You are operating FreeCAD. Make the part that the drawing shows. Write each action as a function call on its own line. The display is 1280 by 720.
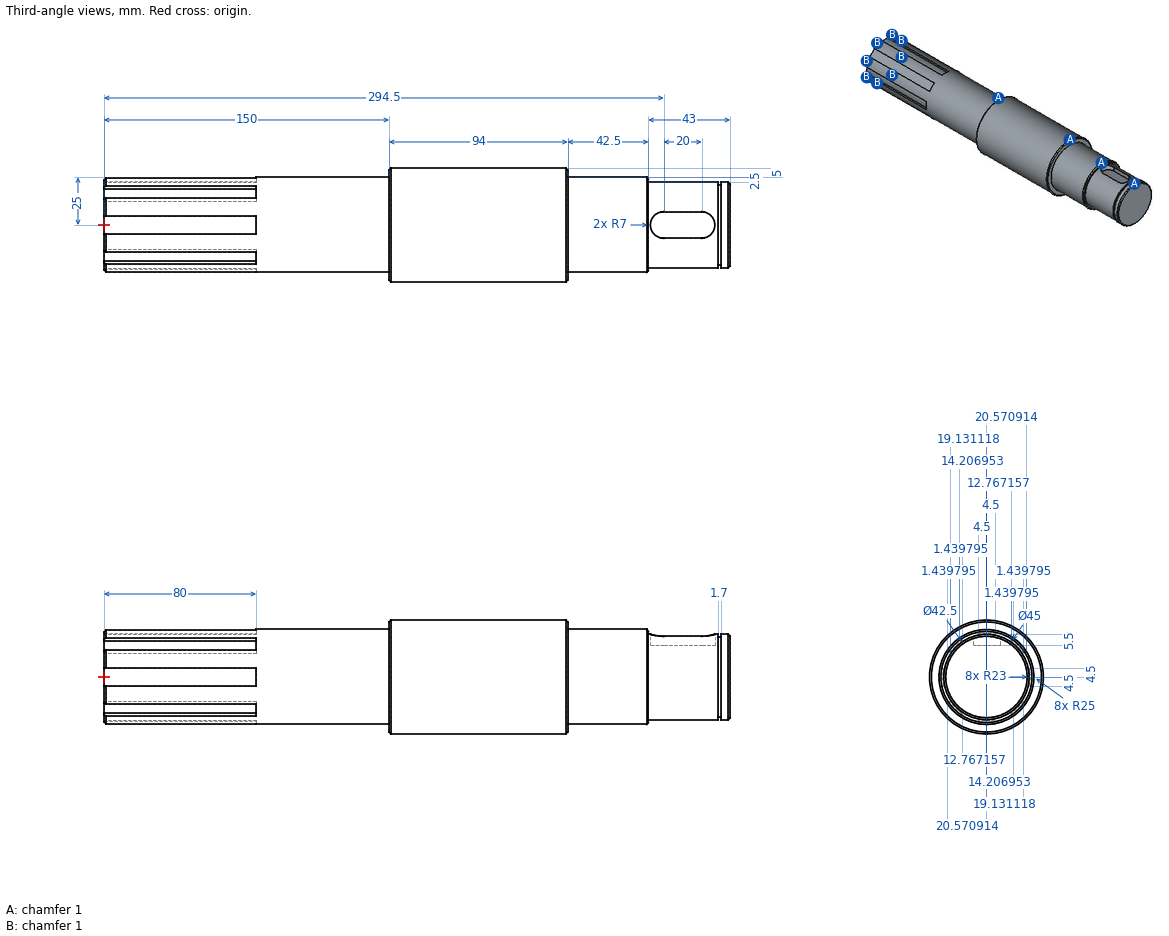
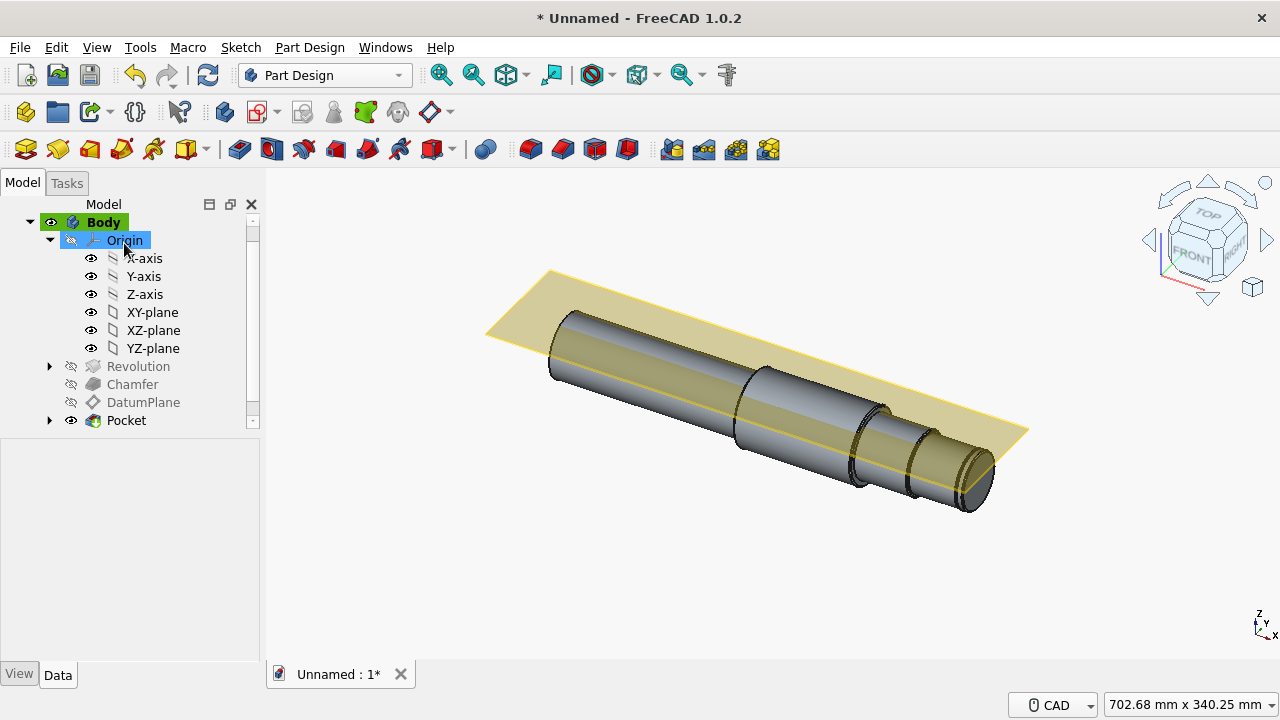
scroll(120, 326, down, 3)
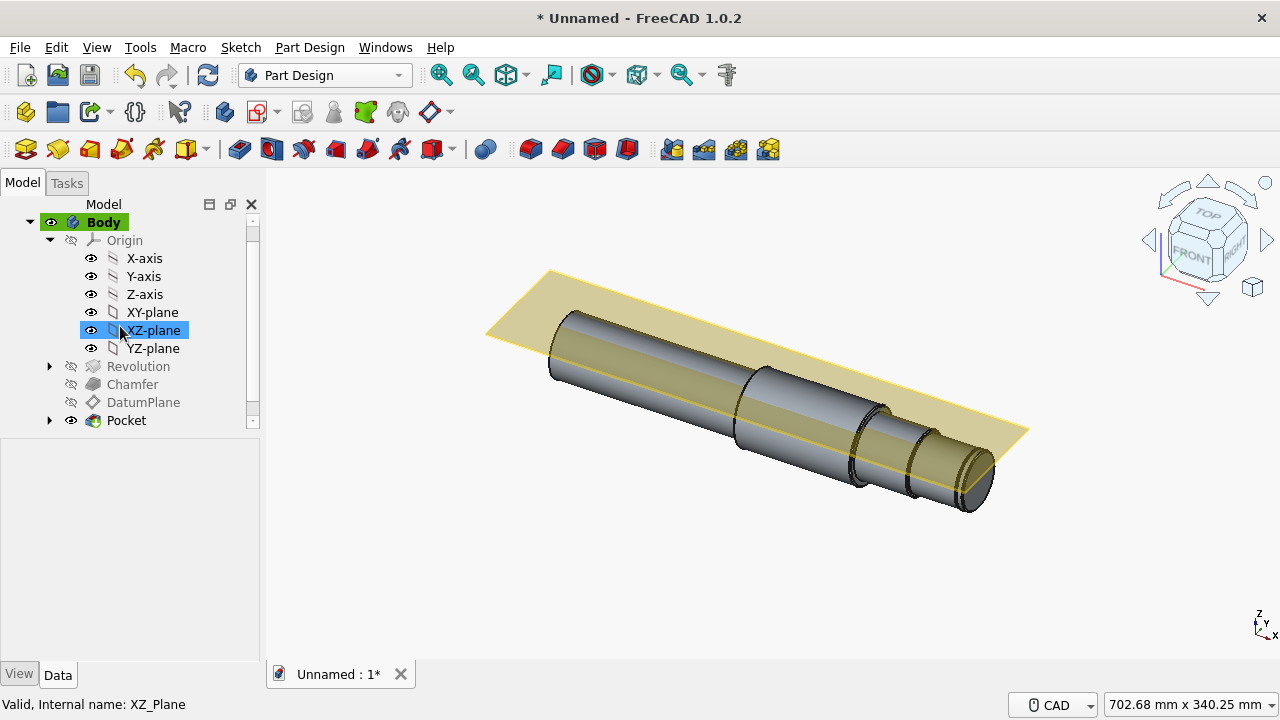
click(116, 420)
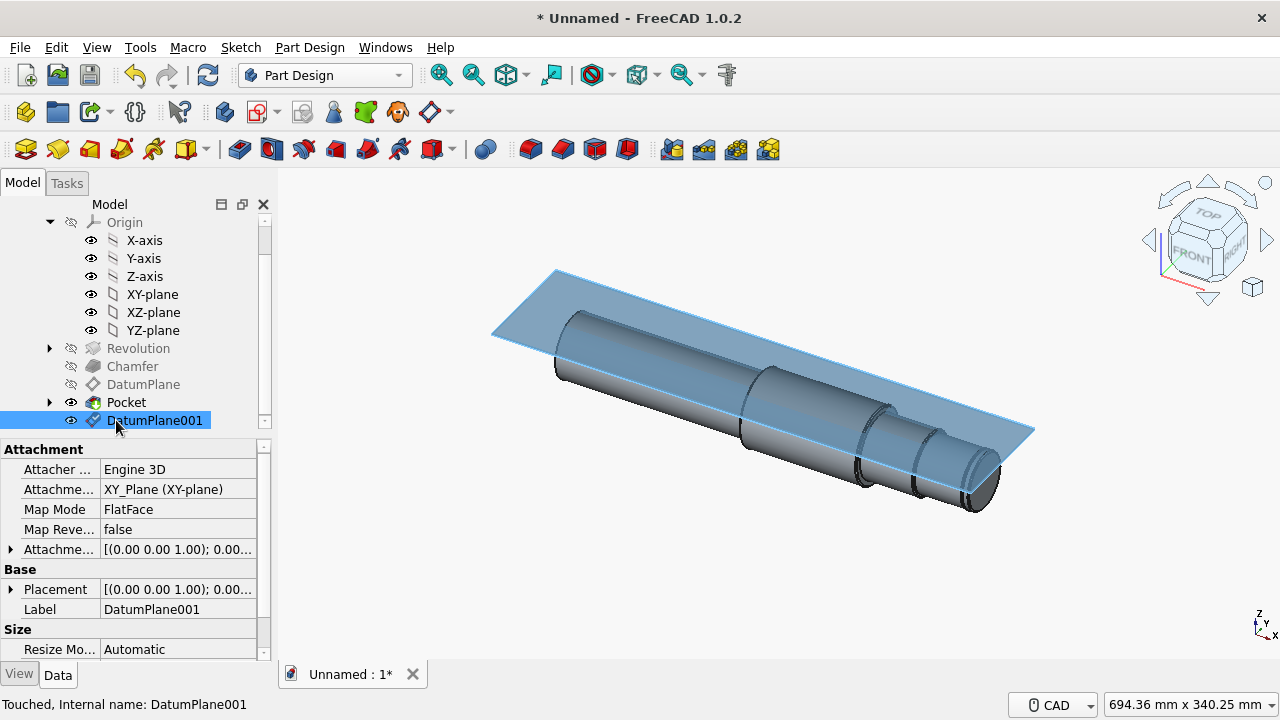
click(258, 112)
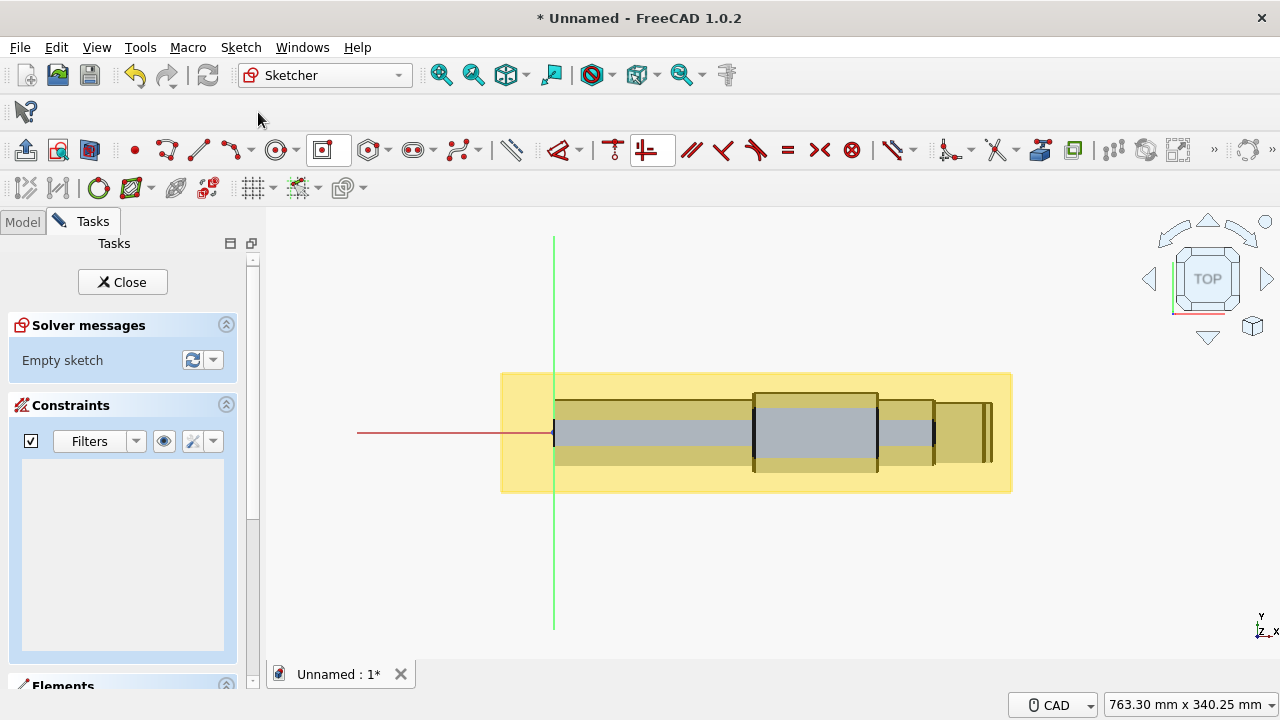
click(90, 150)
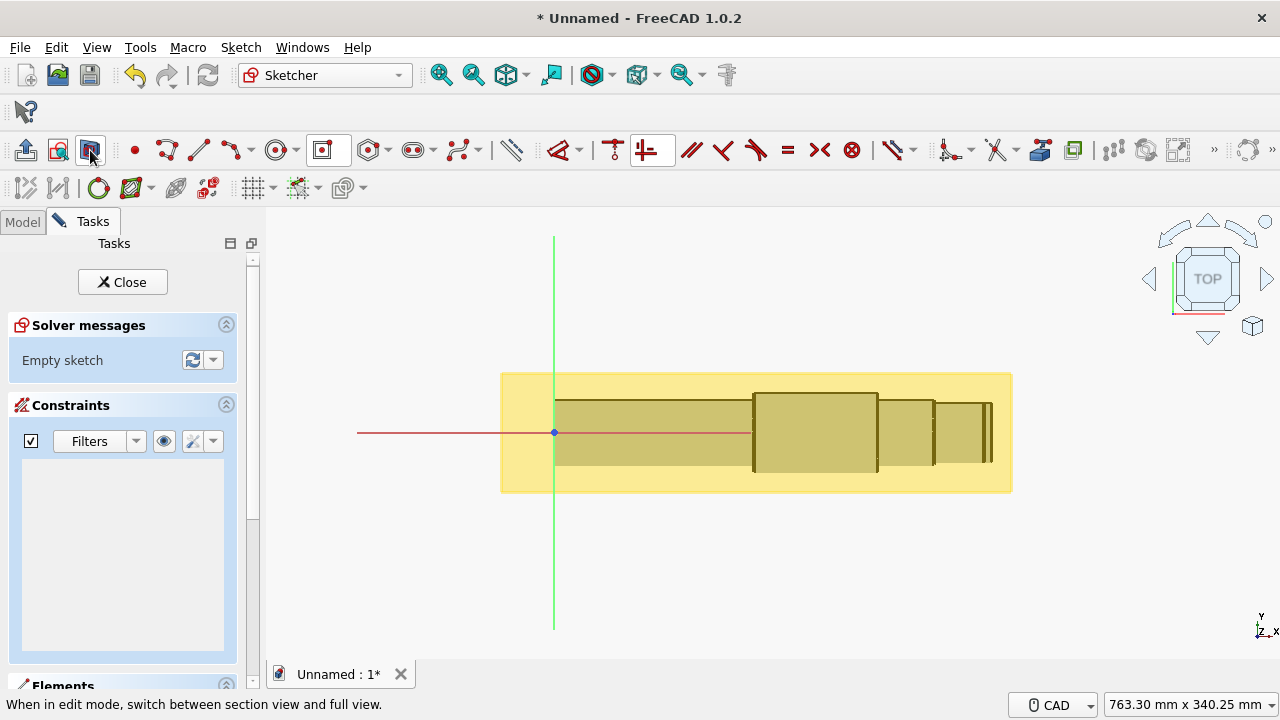
scroll(979, 433, up, 13)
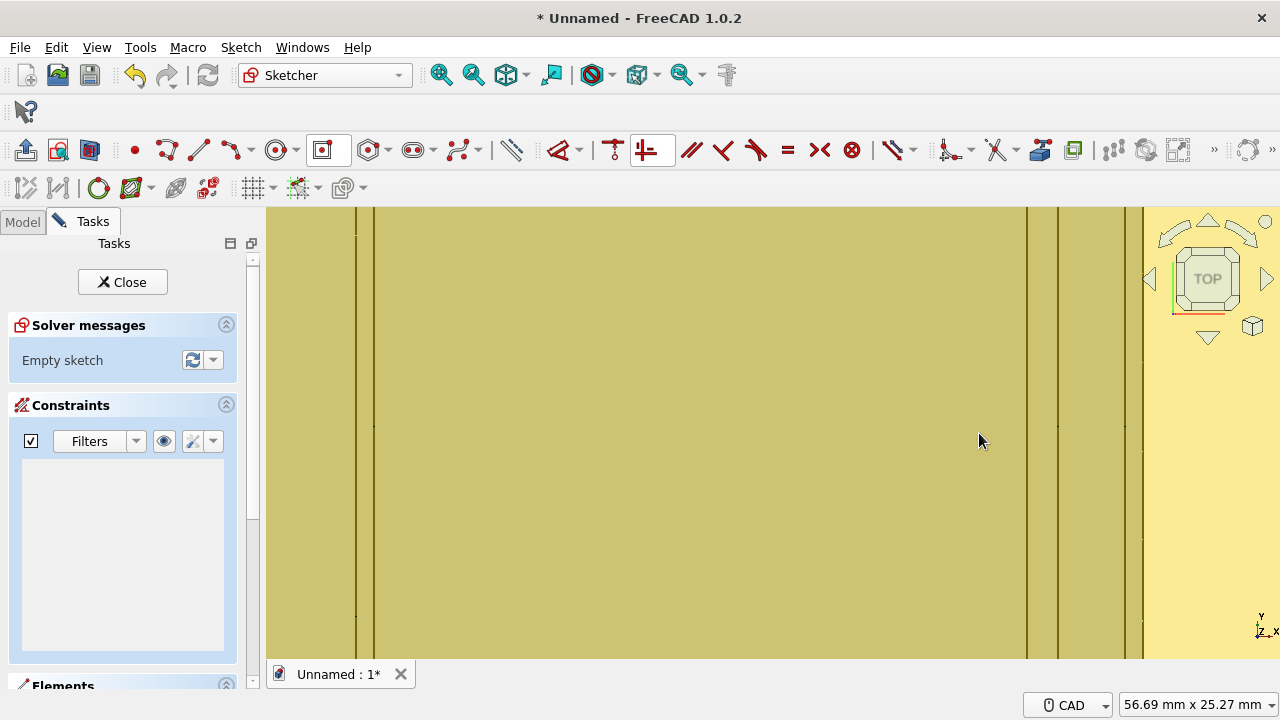
click(414, 150)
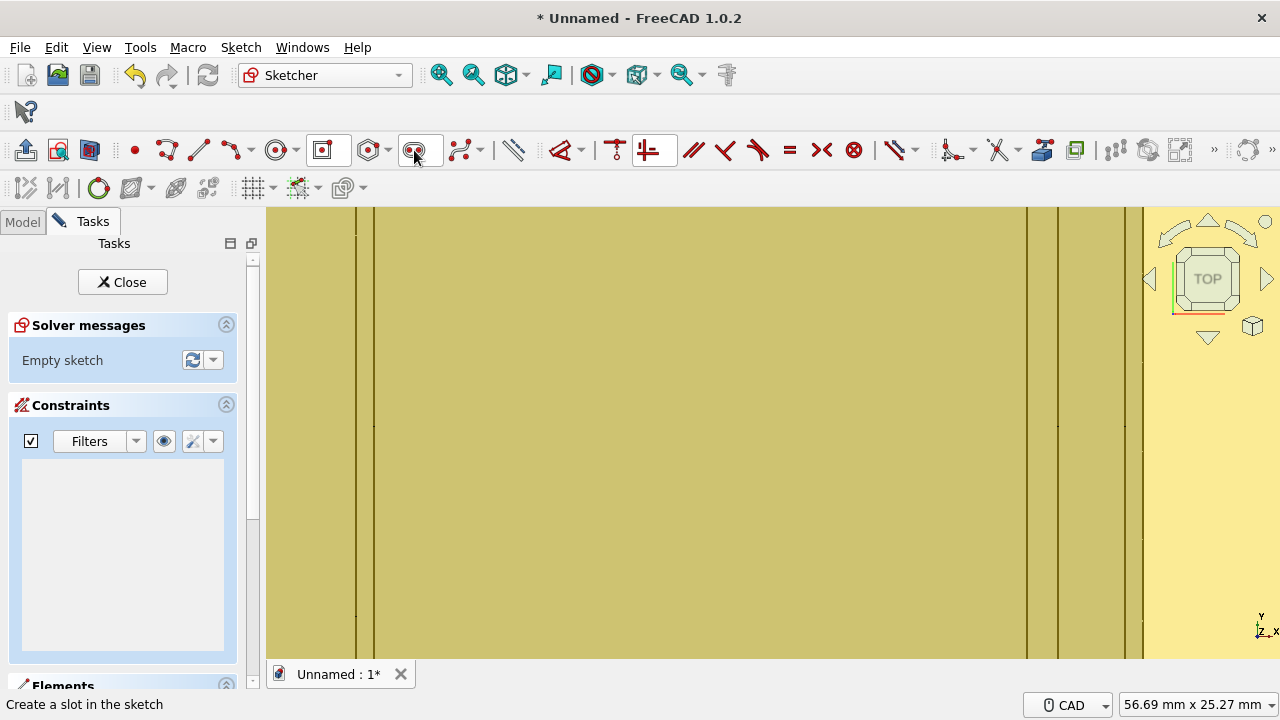
click(517, 427)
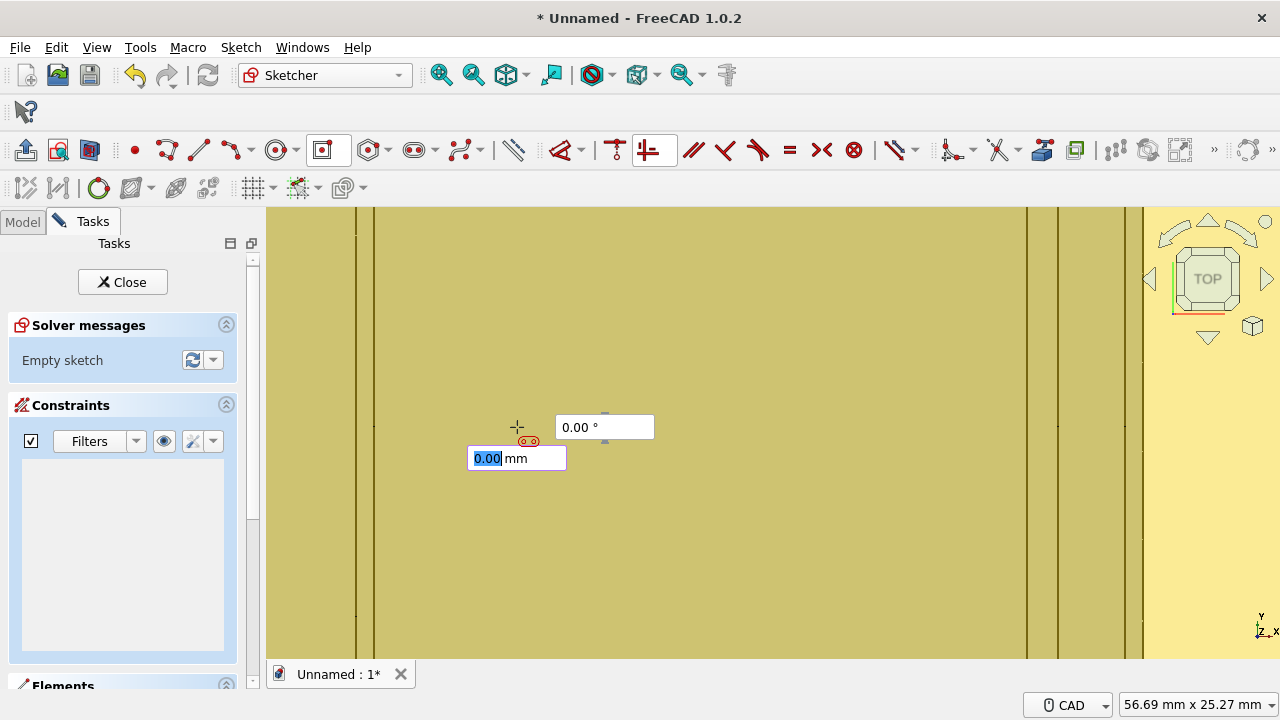
click(875, 418)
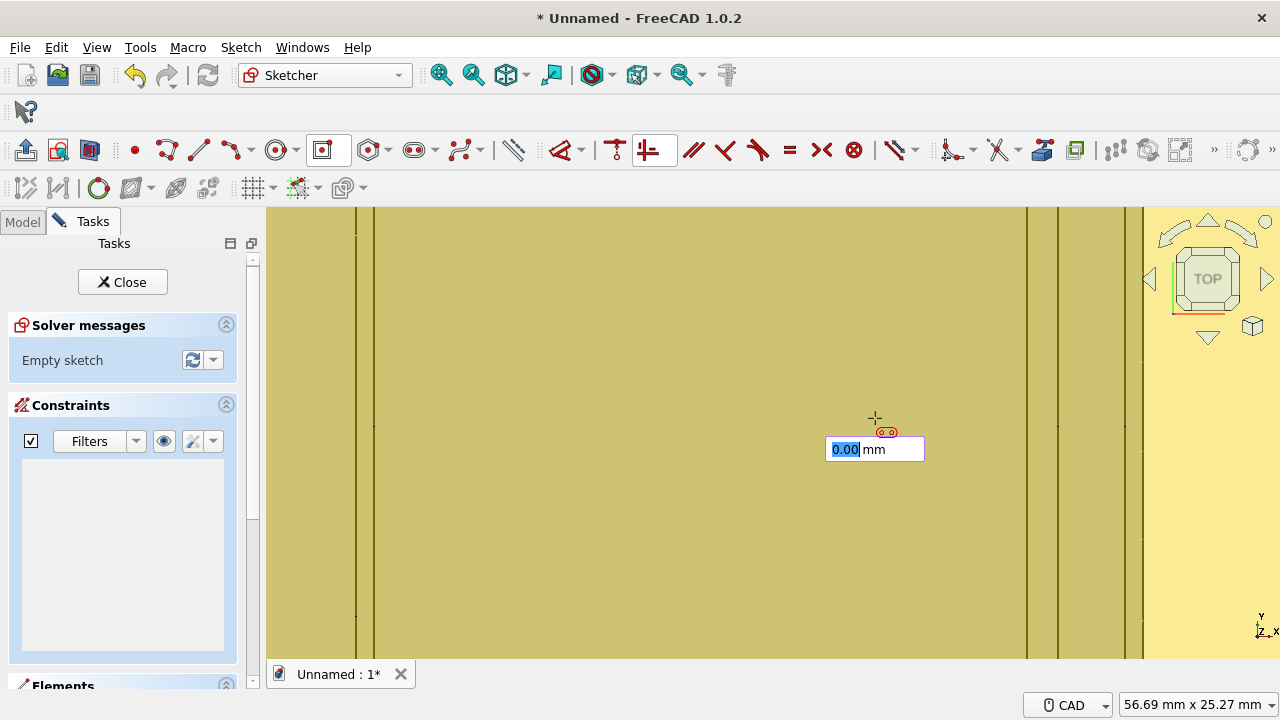
click(696, 302)
key(Escape)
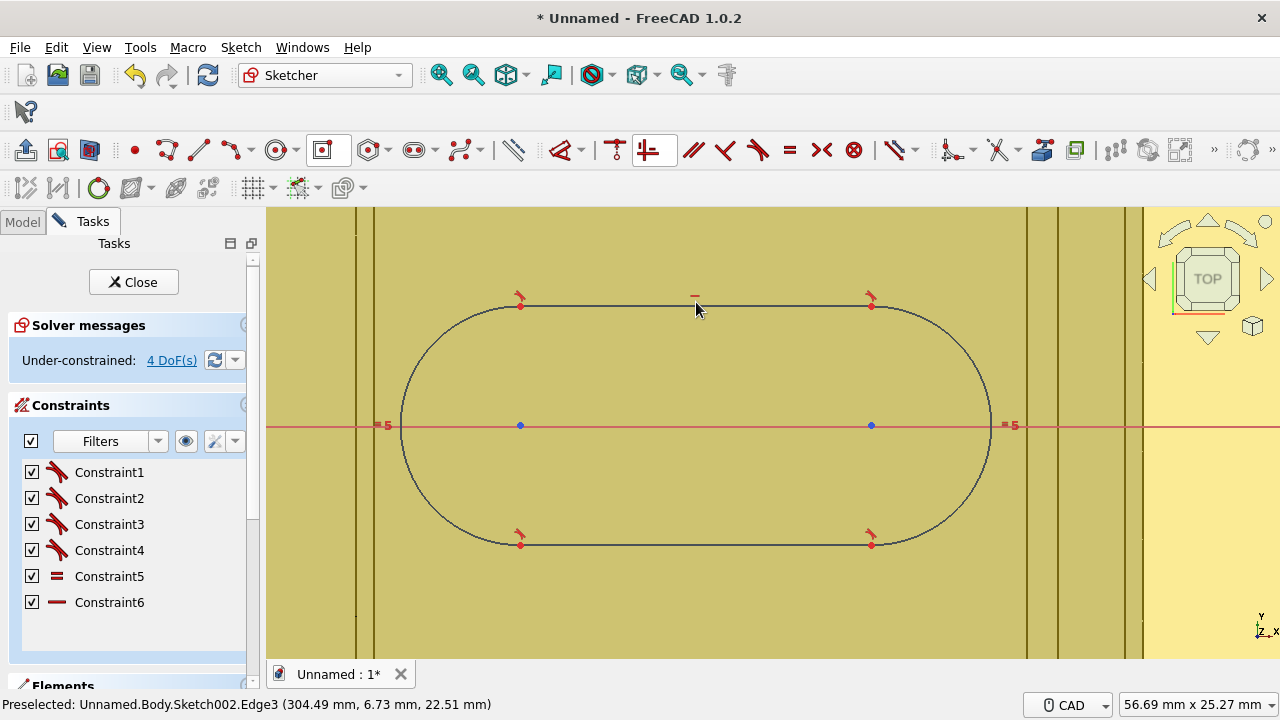
click(520, 426)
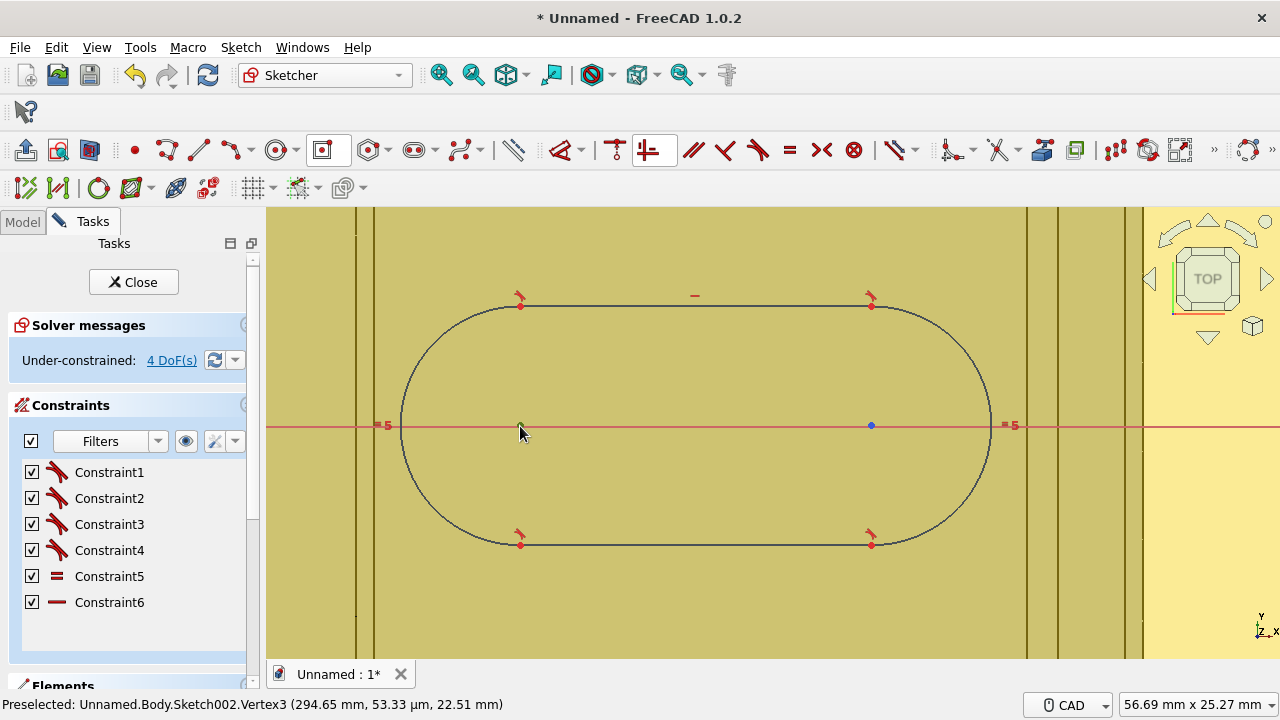
click(353, 427)